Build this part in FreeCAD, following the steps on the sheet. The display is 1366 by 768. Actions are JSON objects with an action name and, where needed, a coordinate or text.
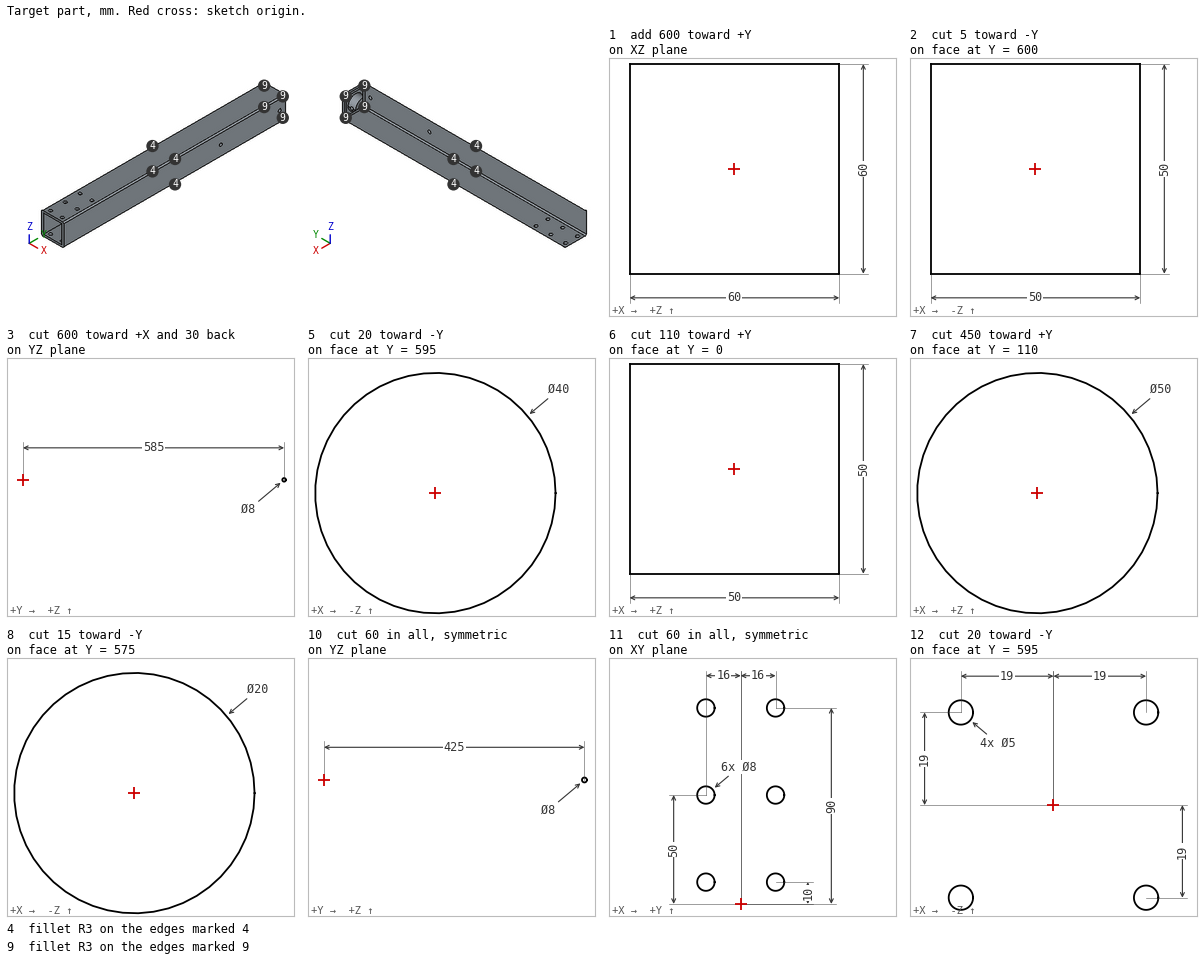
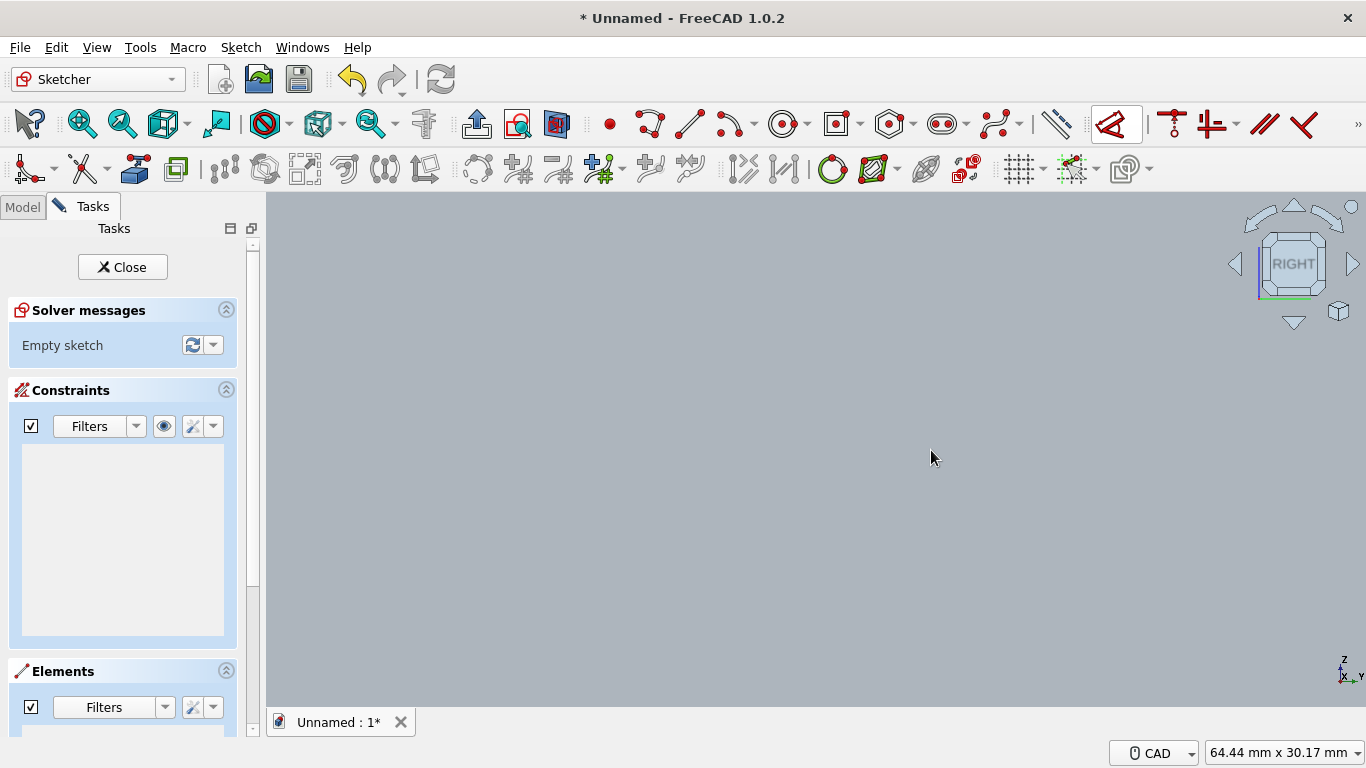
{"action": "scroll", "coordinate": [740, 415], "scroll_direction": "up", "scroll_amount": 4}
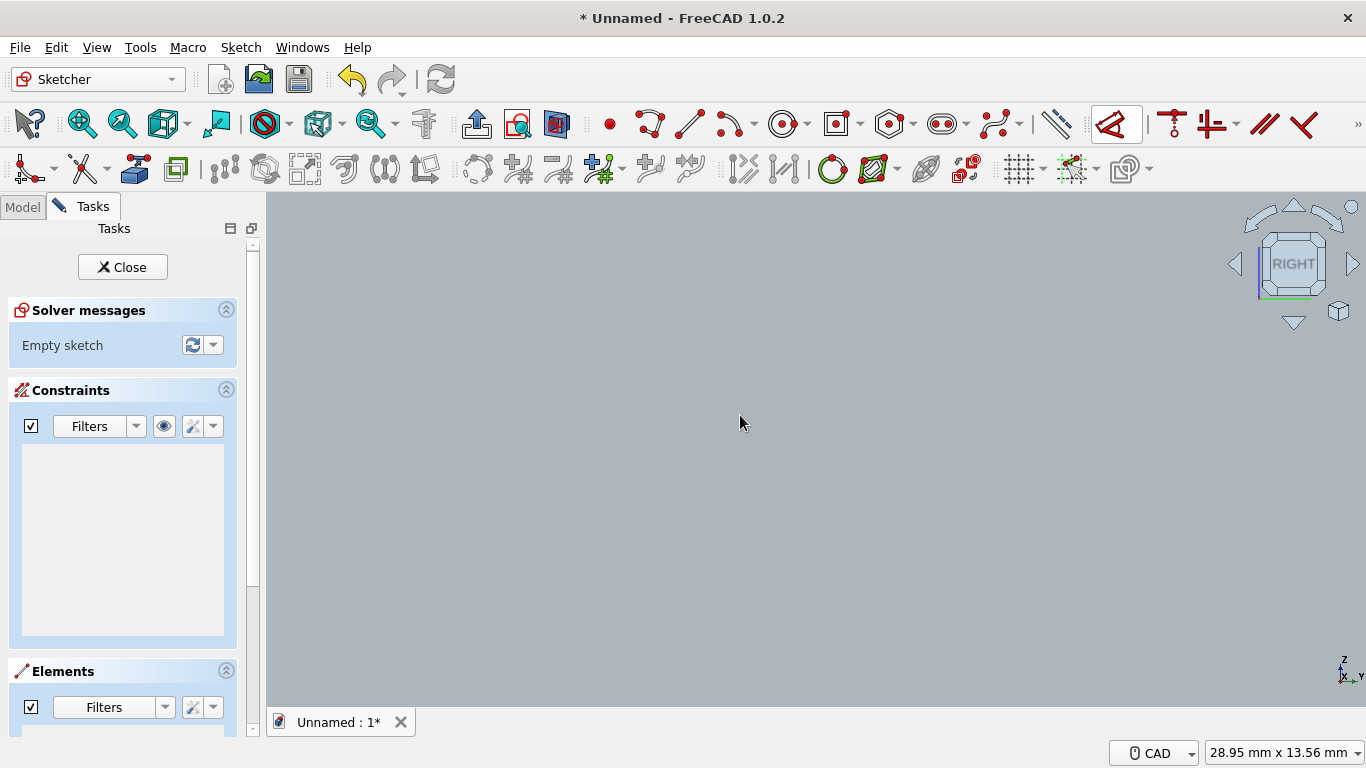
{"action": "left_click", "coordinate": [784, 124]}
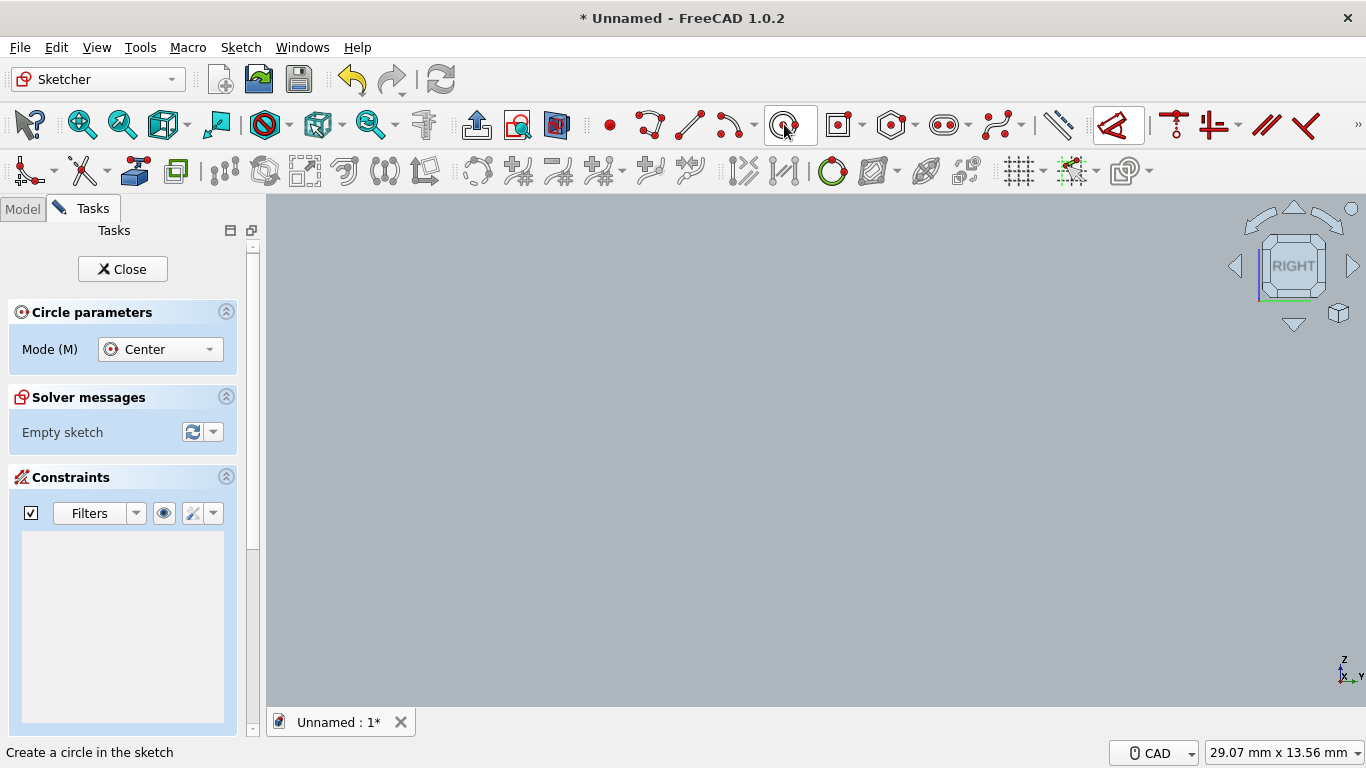
{"action": "left_click", "coordinate": [747, 450]}
{"action": "mouse_move", "coordinate": [854, 343]}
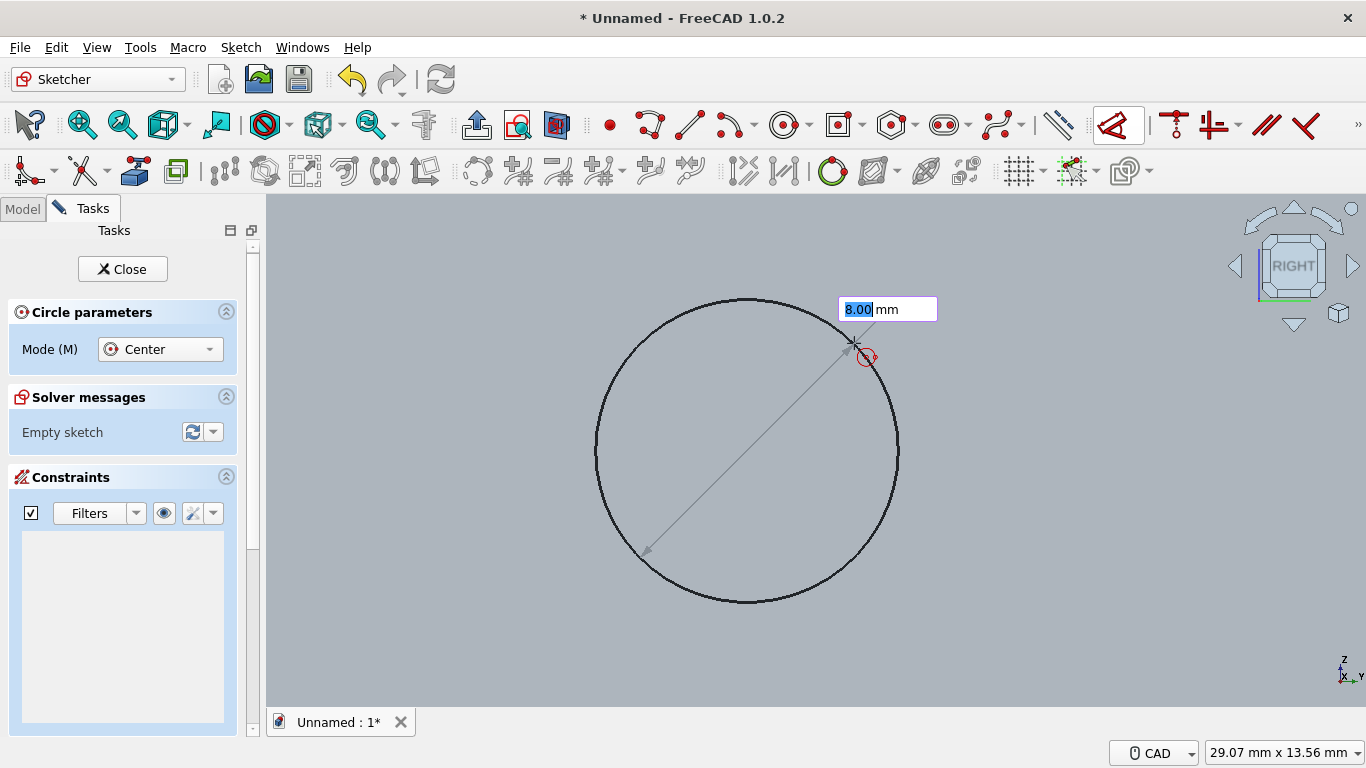
{"action": "type", "text": "8"}
{"action": "key", "text": "Return"}
{"action": "key", "text": "Escape"}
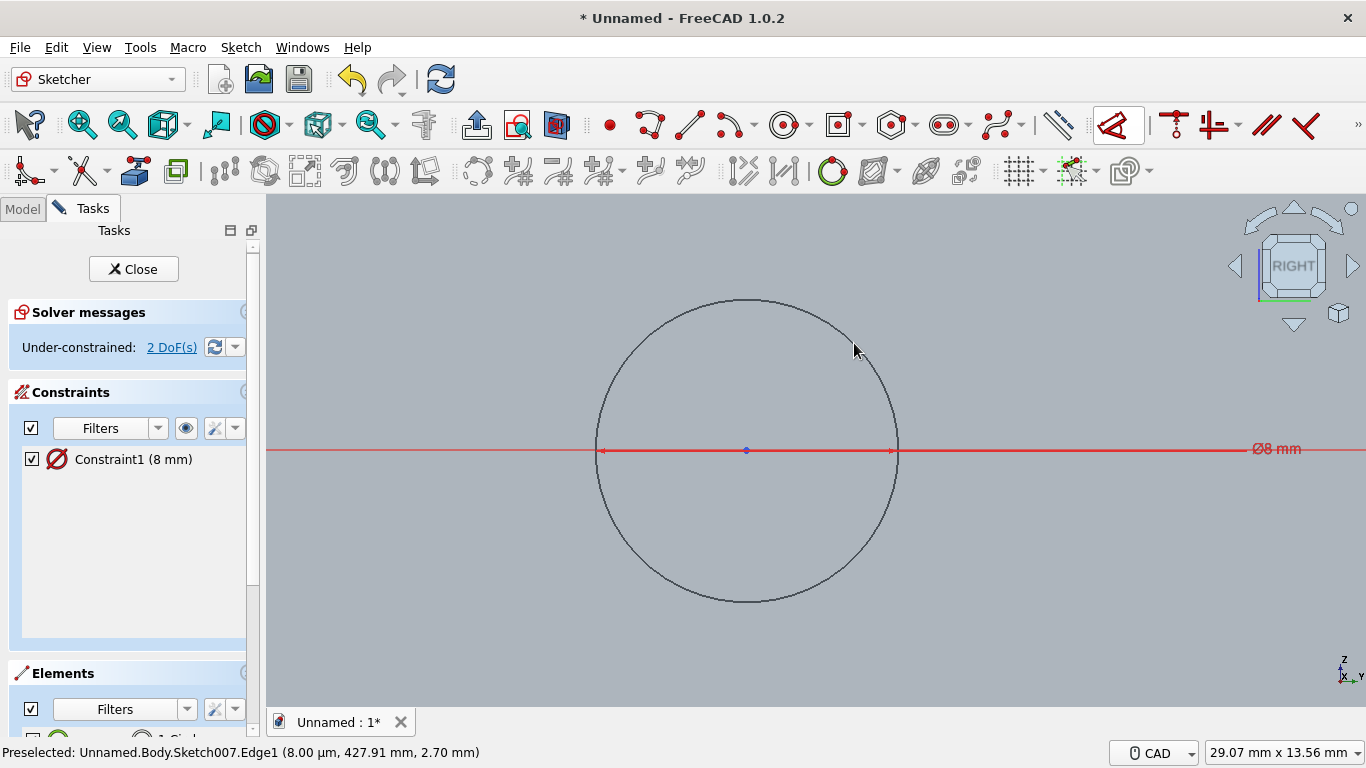
{"action": "left_click", "coordinate": [747, 451]}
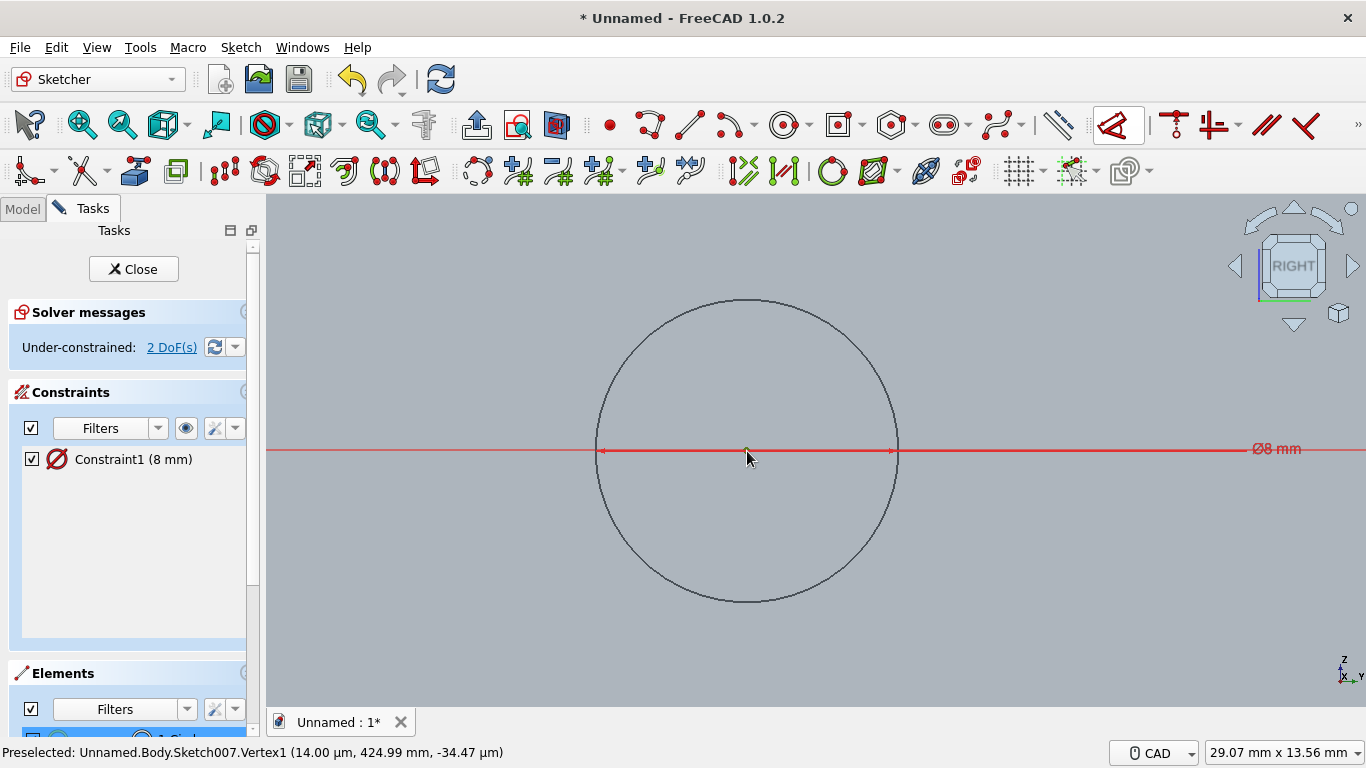
{"action": "left_click", "coordinate": [359, 450]}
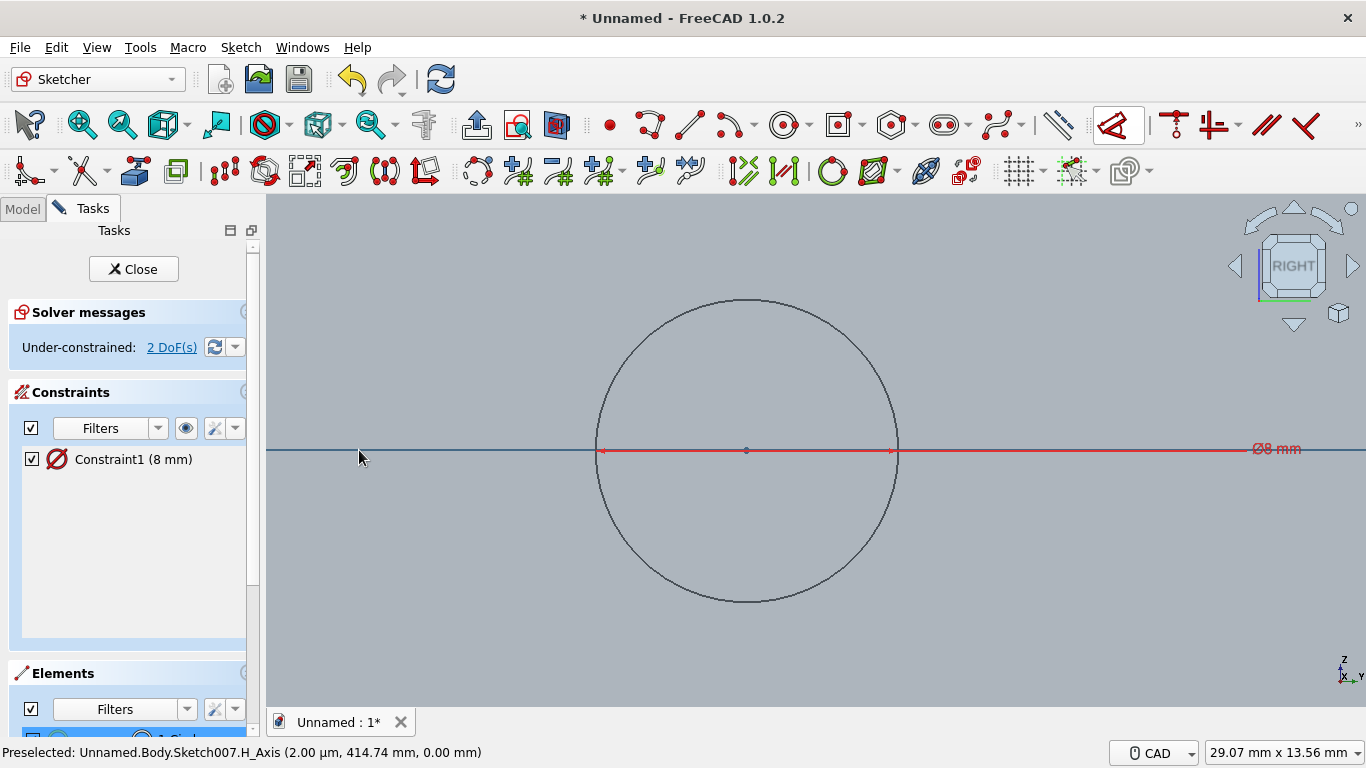
{"action": "key", "text": "c"}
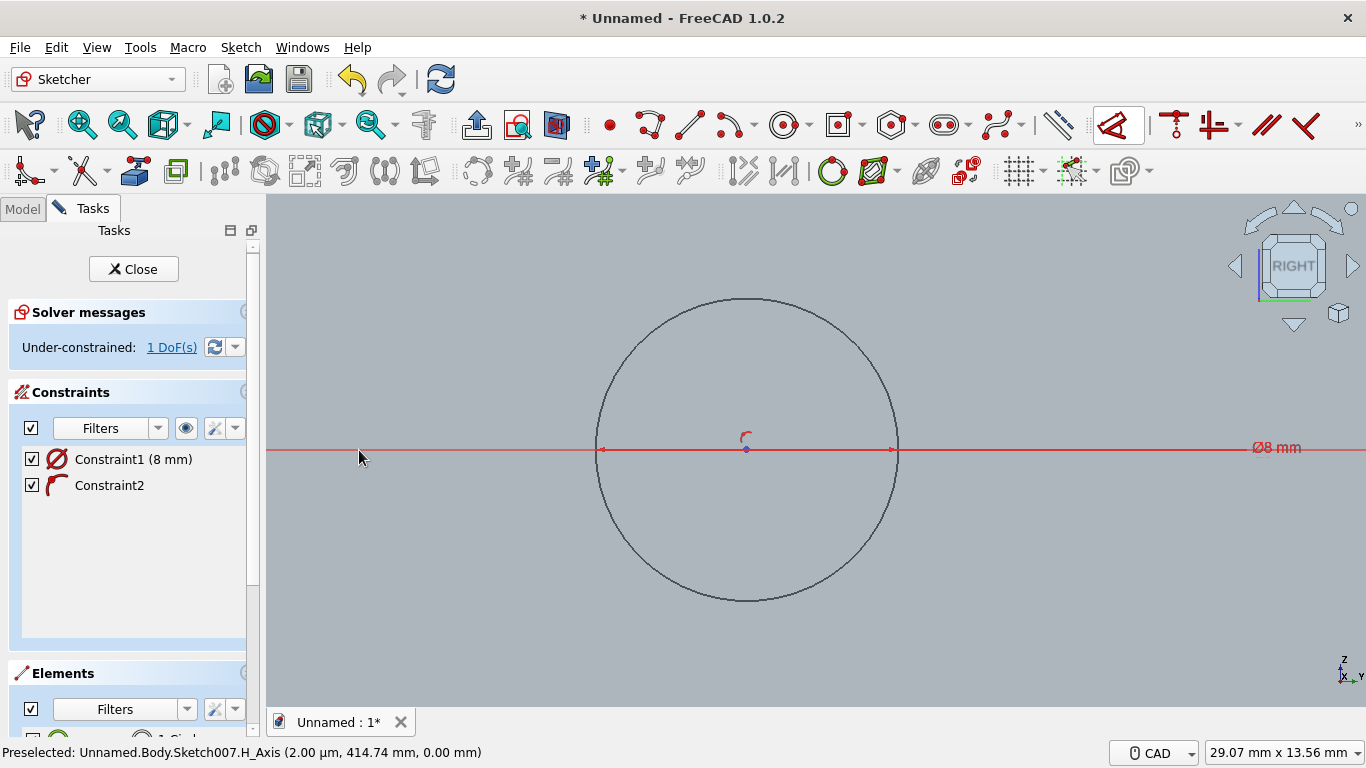
{"action": "left_click", "coordinate": [747, 450]}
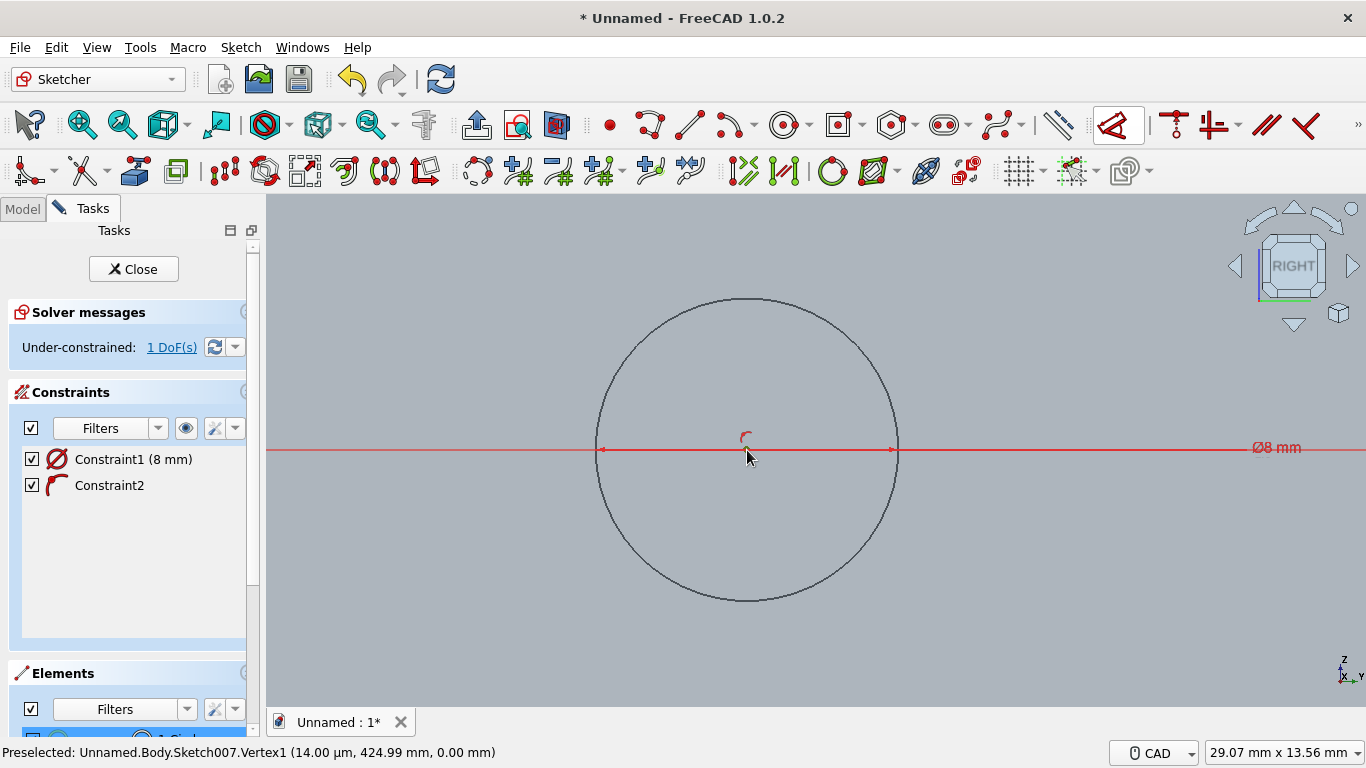
{"action": "key", "text": "l"}